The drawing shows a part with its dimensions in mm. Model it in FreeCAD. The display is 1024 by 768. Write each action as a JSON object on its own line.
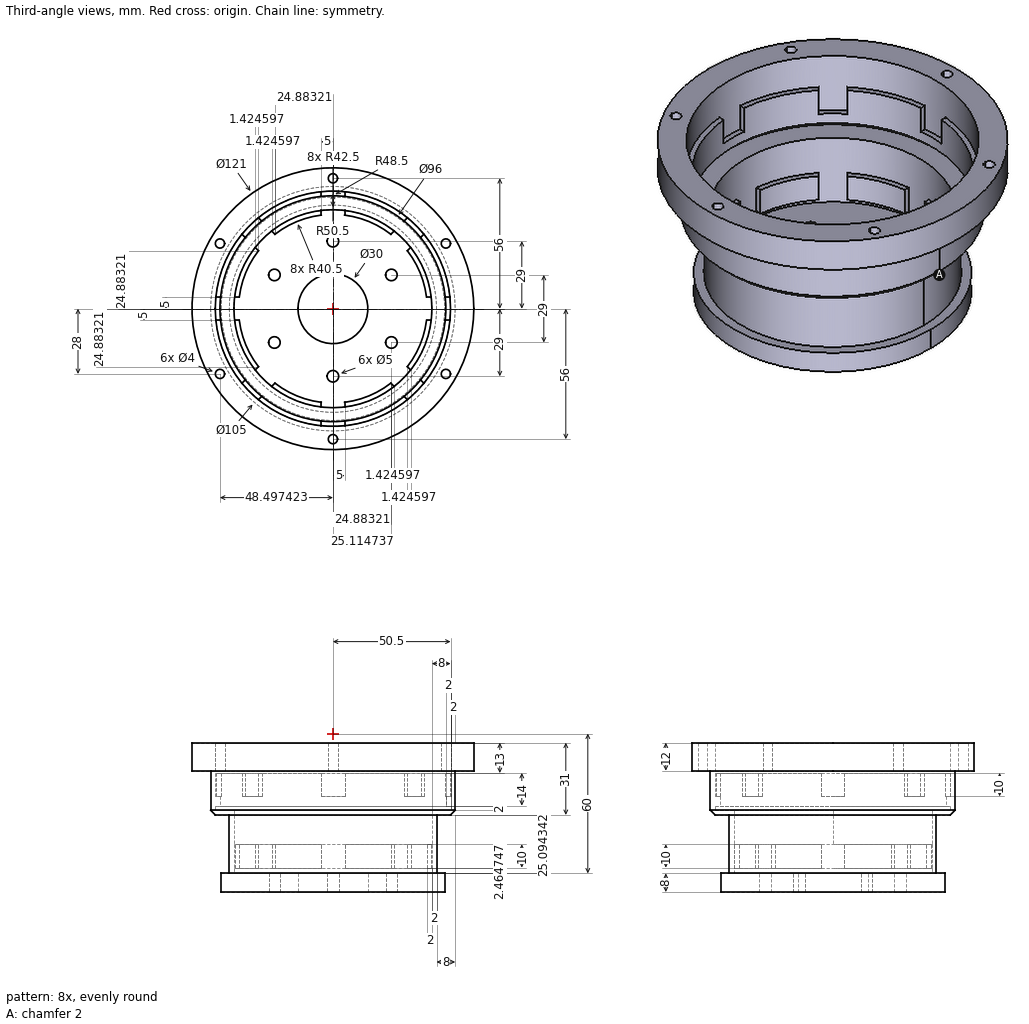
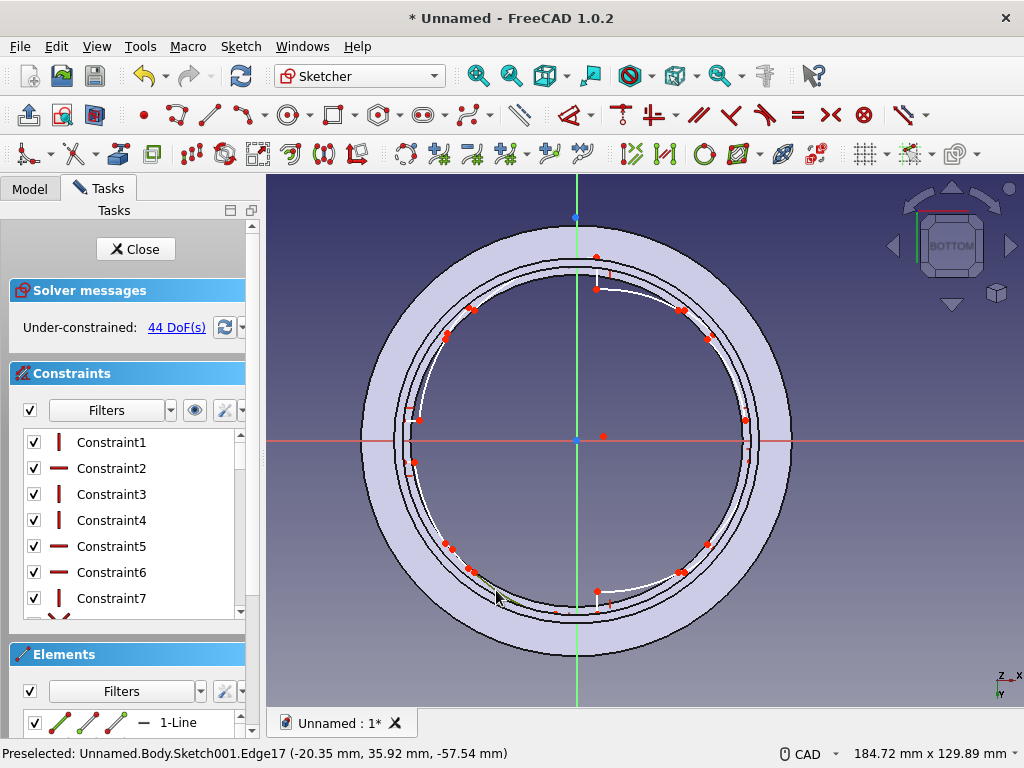
{"action": "left_click", "coordinate": [577, 615]}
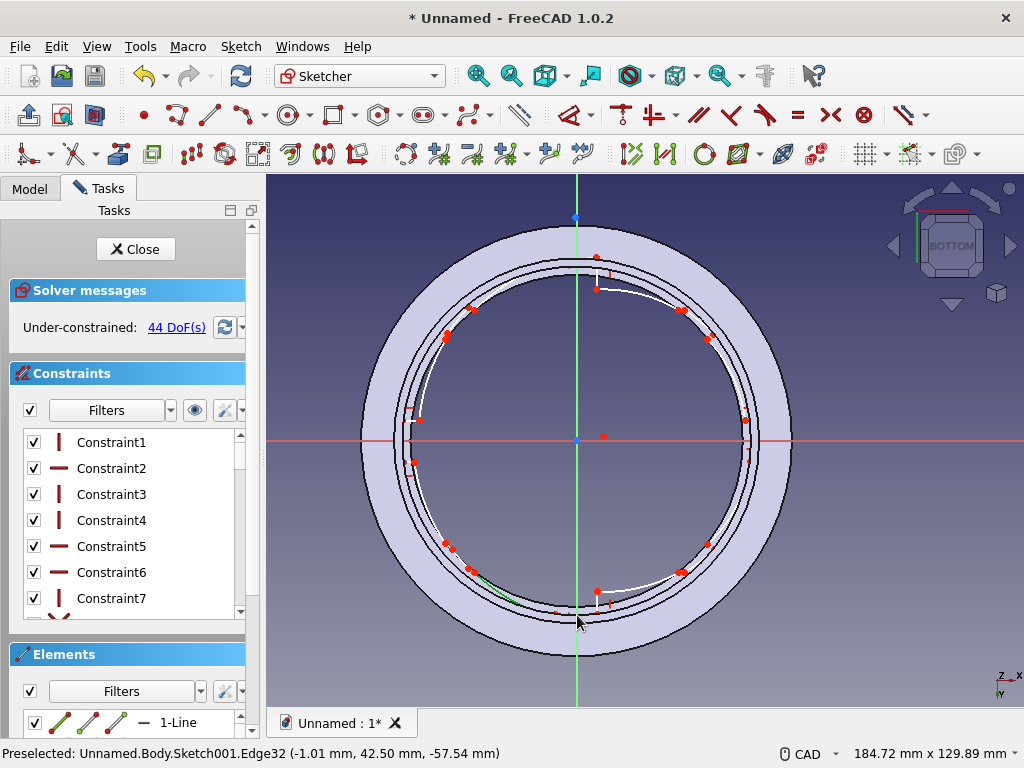
{"action": "left_click", "coordinate": [621, 116]}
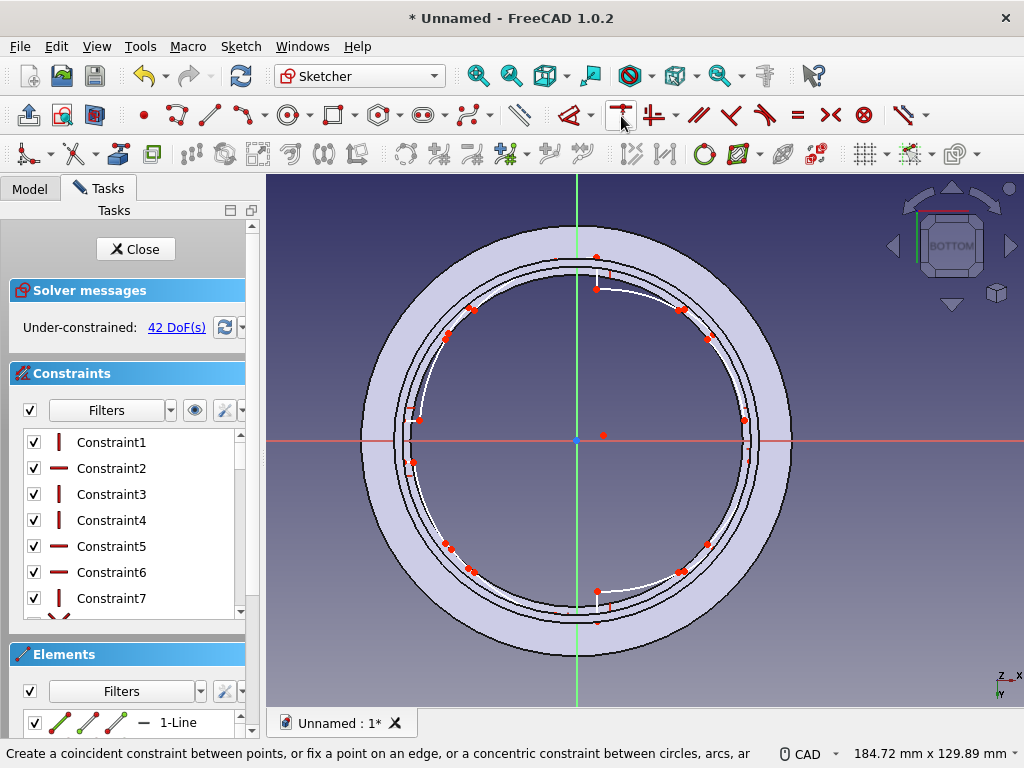
{"action": "left_click_drag", "start_coordinate": [567, 425], "coordinate": [614, 451]}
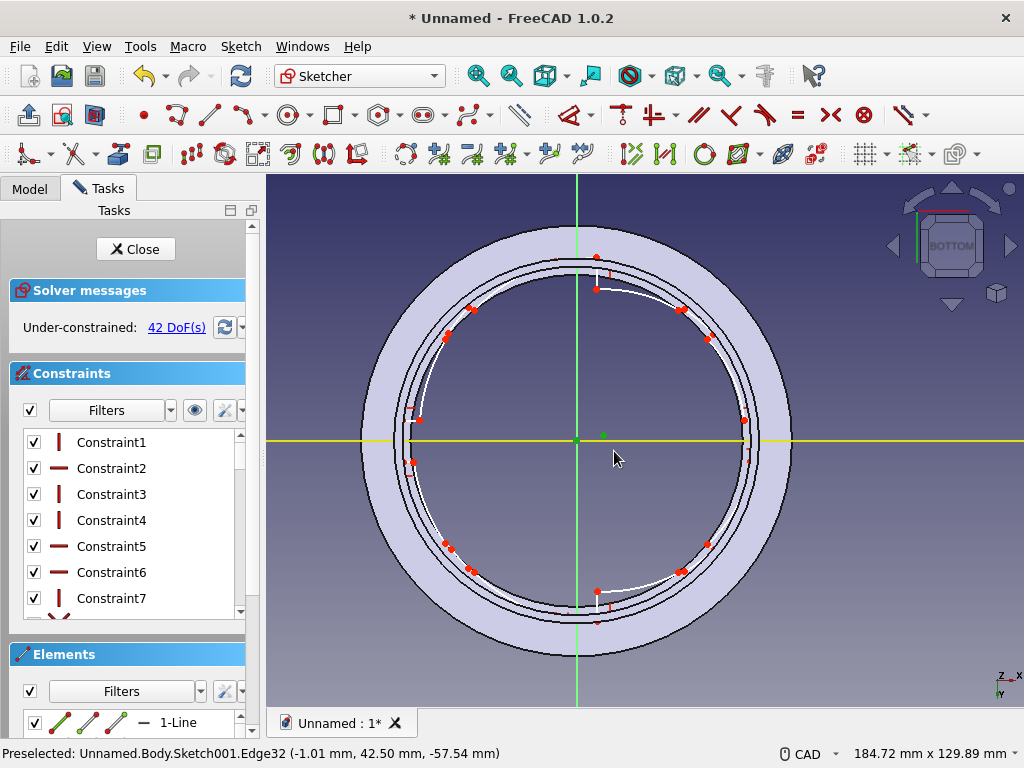
{"action": "key", "text": "c"}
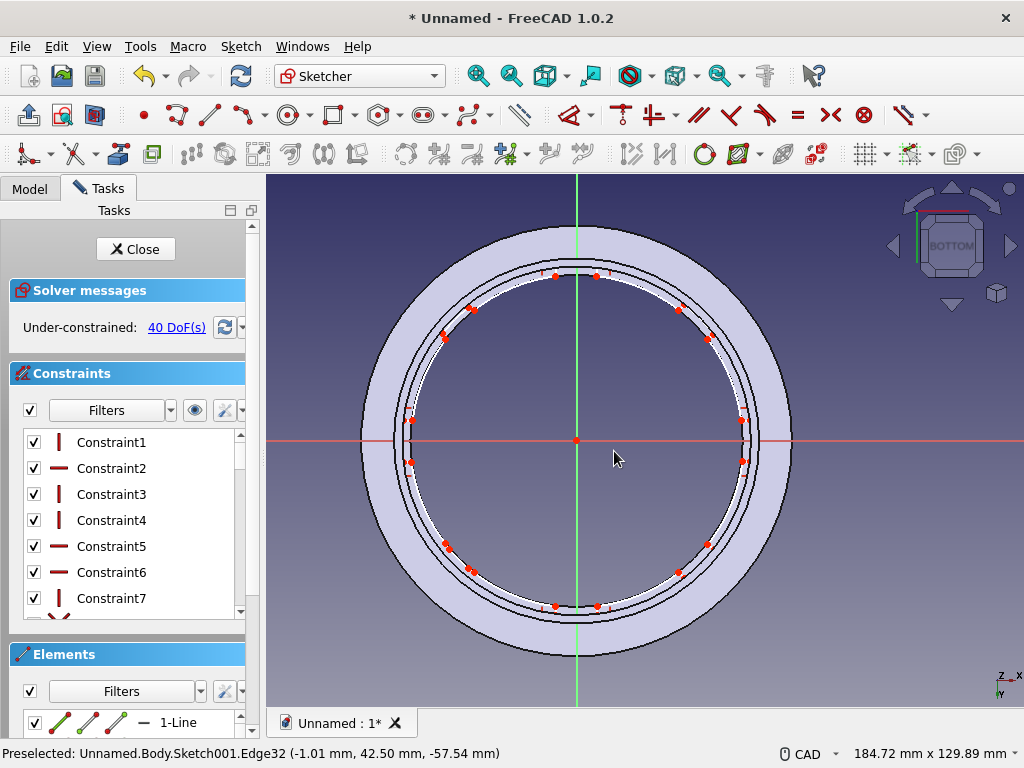
{"action": "left_click", "coordinate": [497, 587]}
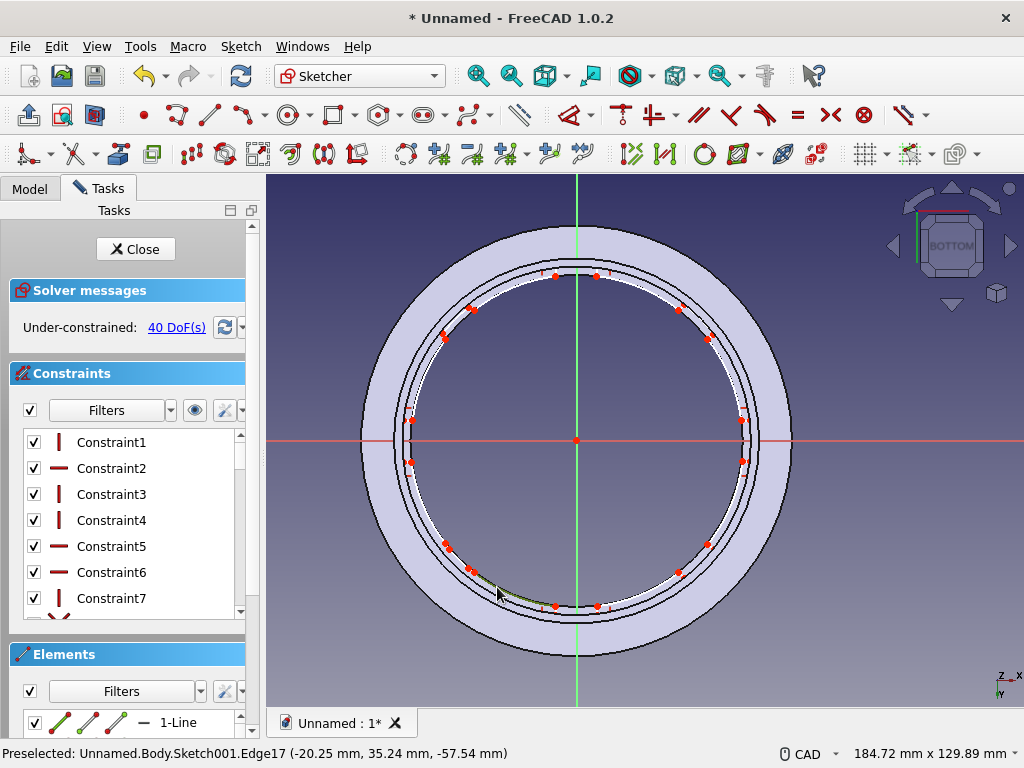
{"action": "left_click", "coordinate": [417, 488]}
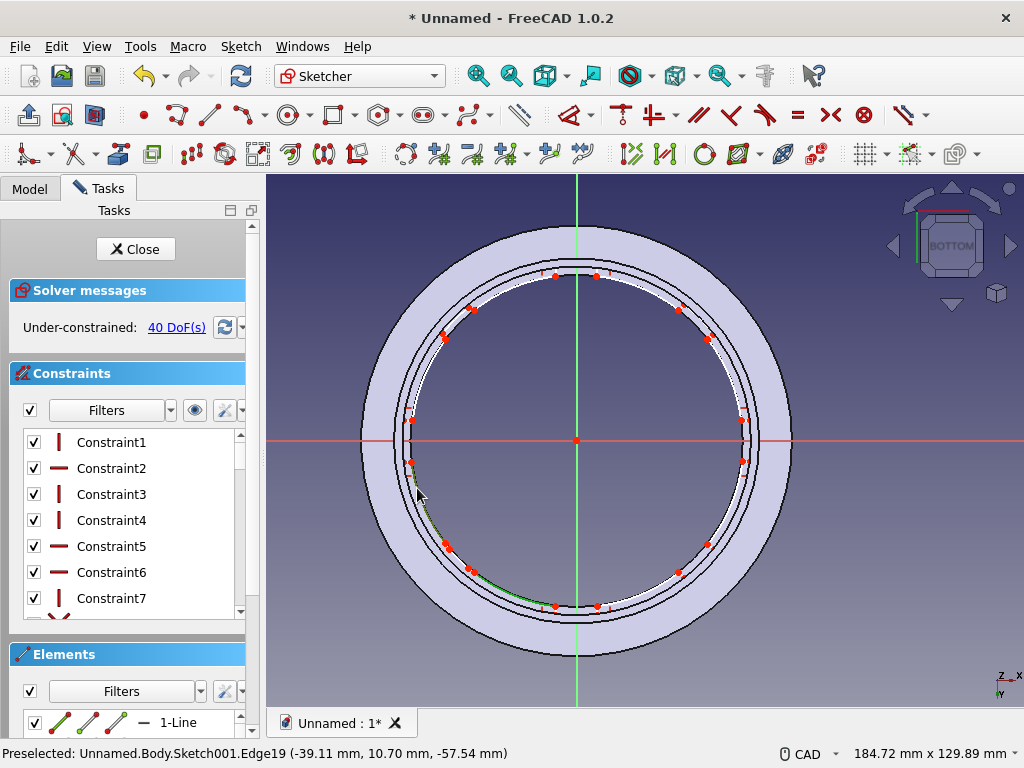
{"action": "left_click", "coordinate": [431, 362]}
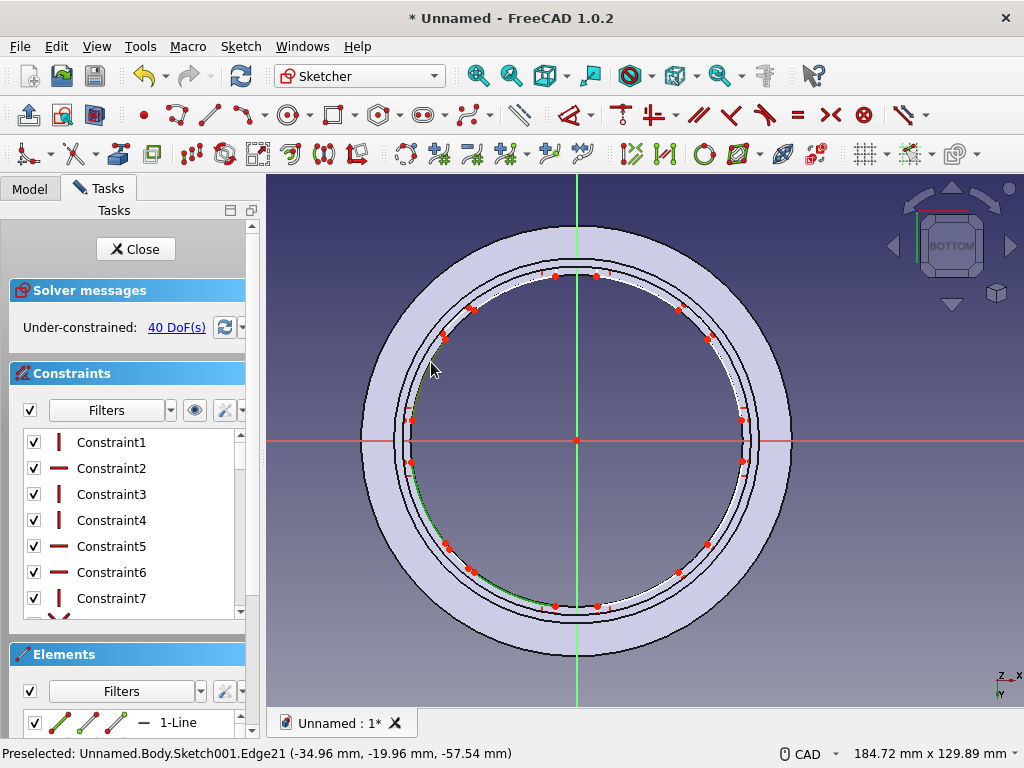
{"action": "left_click", "coordinate": [530, 282]}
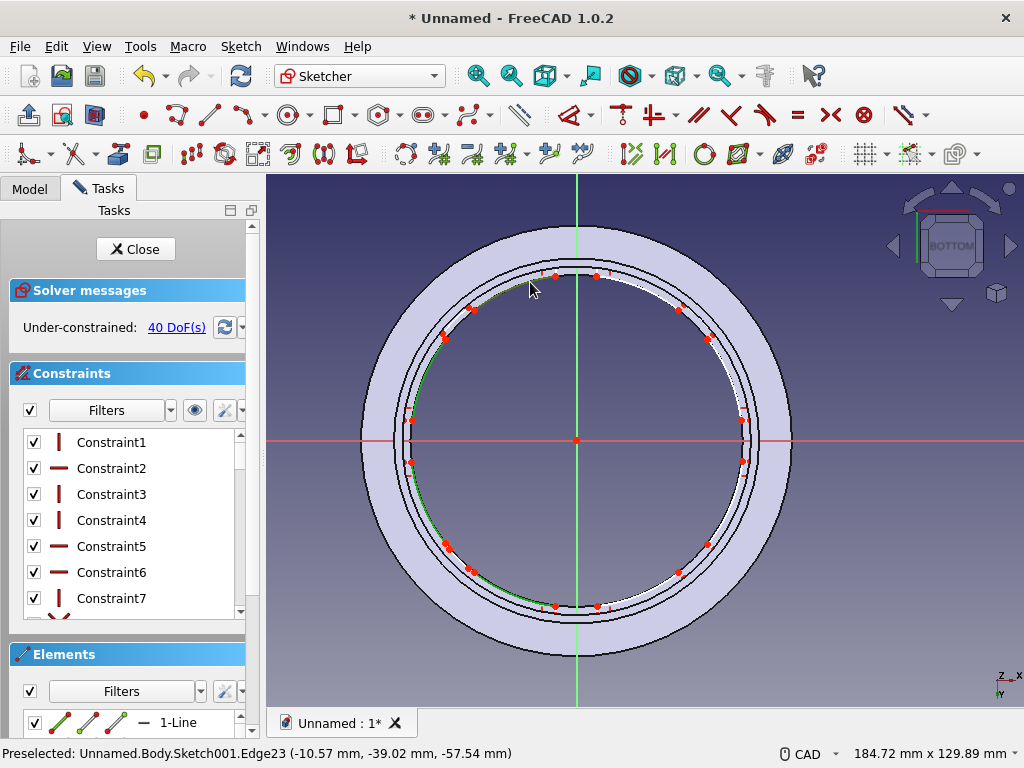
{"action": "left_click", "coordinate": [656, 295]}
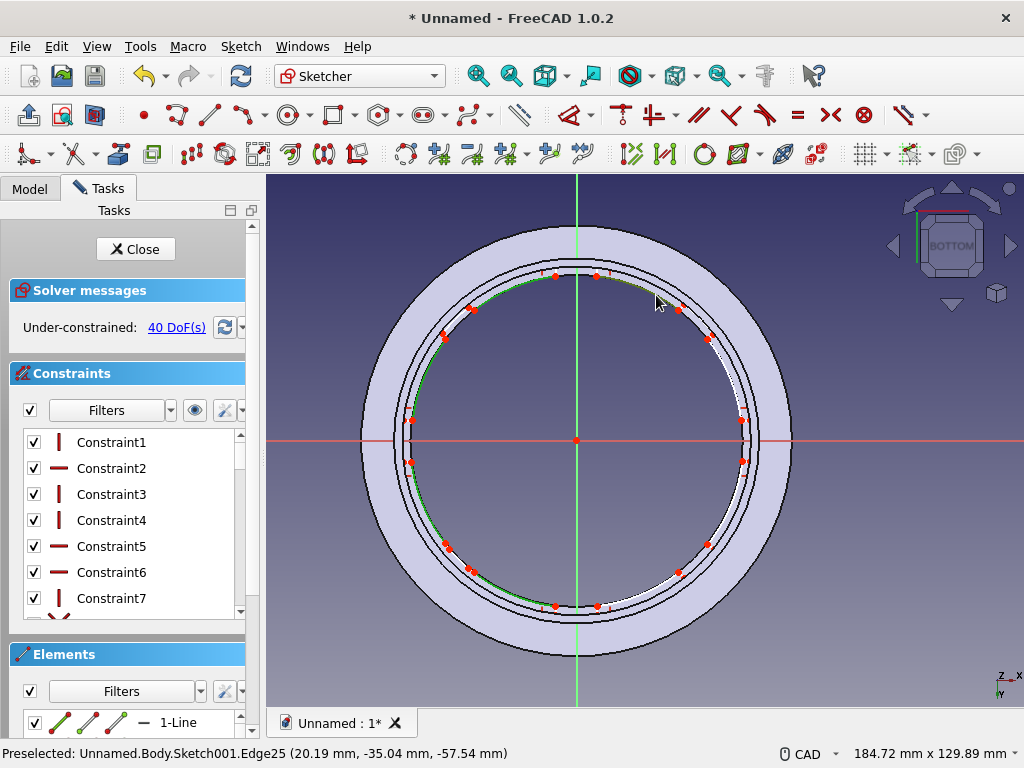
{"action": "left_click", "coordinate": [736, 395]}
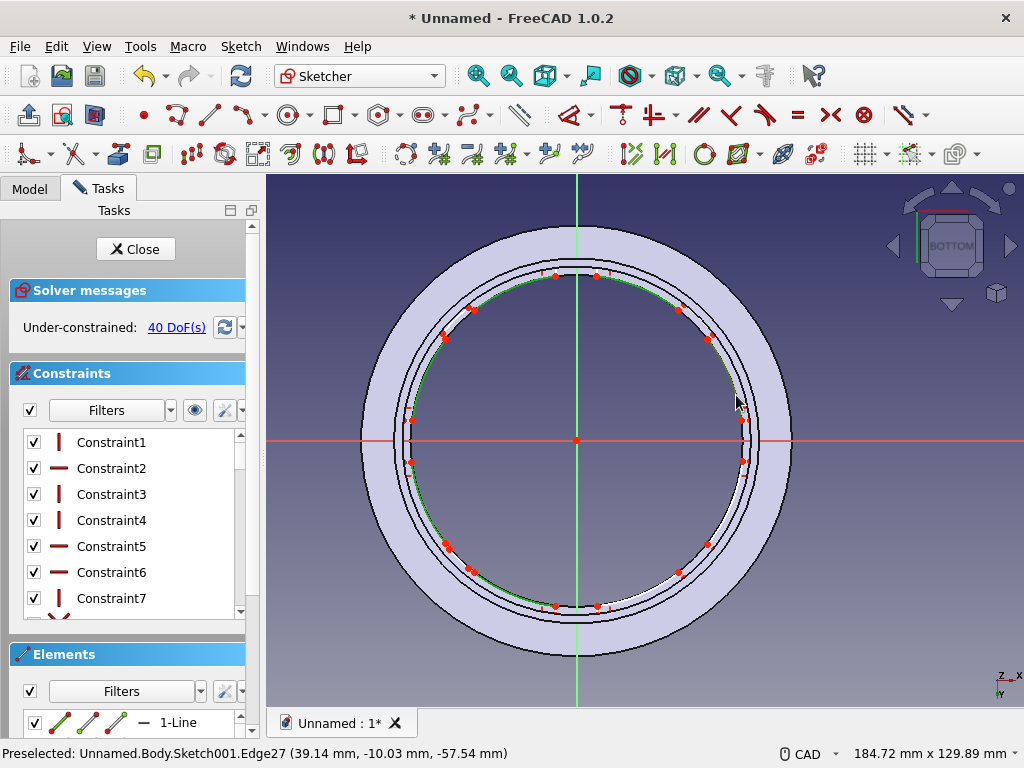
{"action": "left_click", "coordinate": [723, 522]}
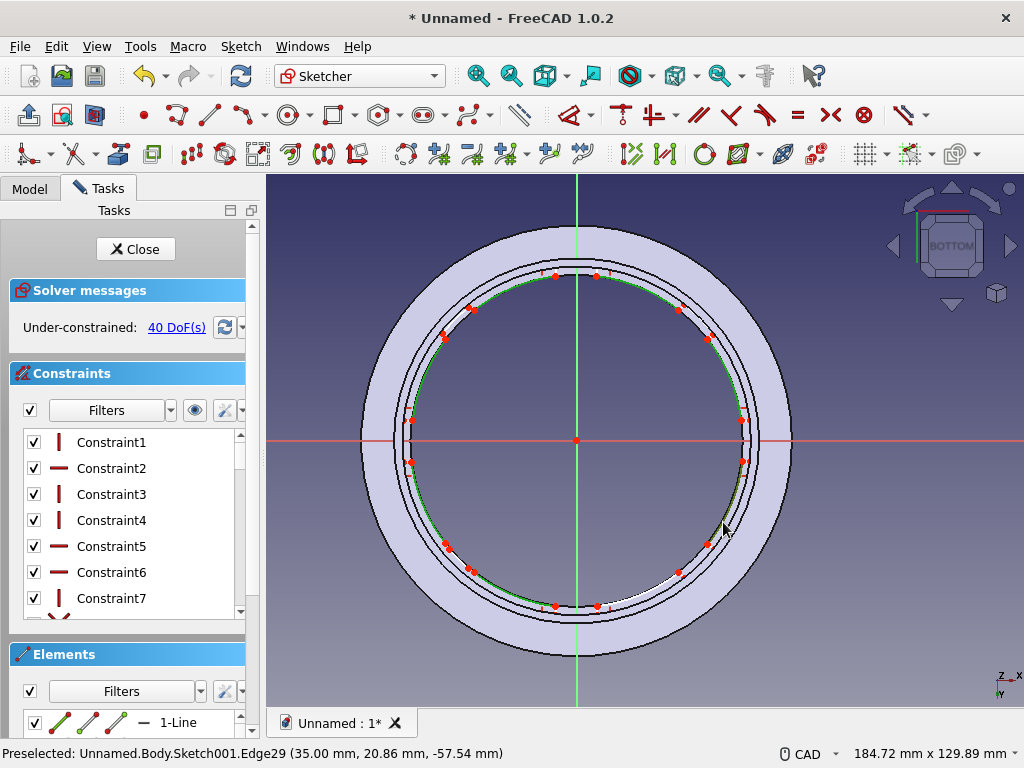
{"action": "left_click", "coordinate": [623, 601]}